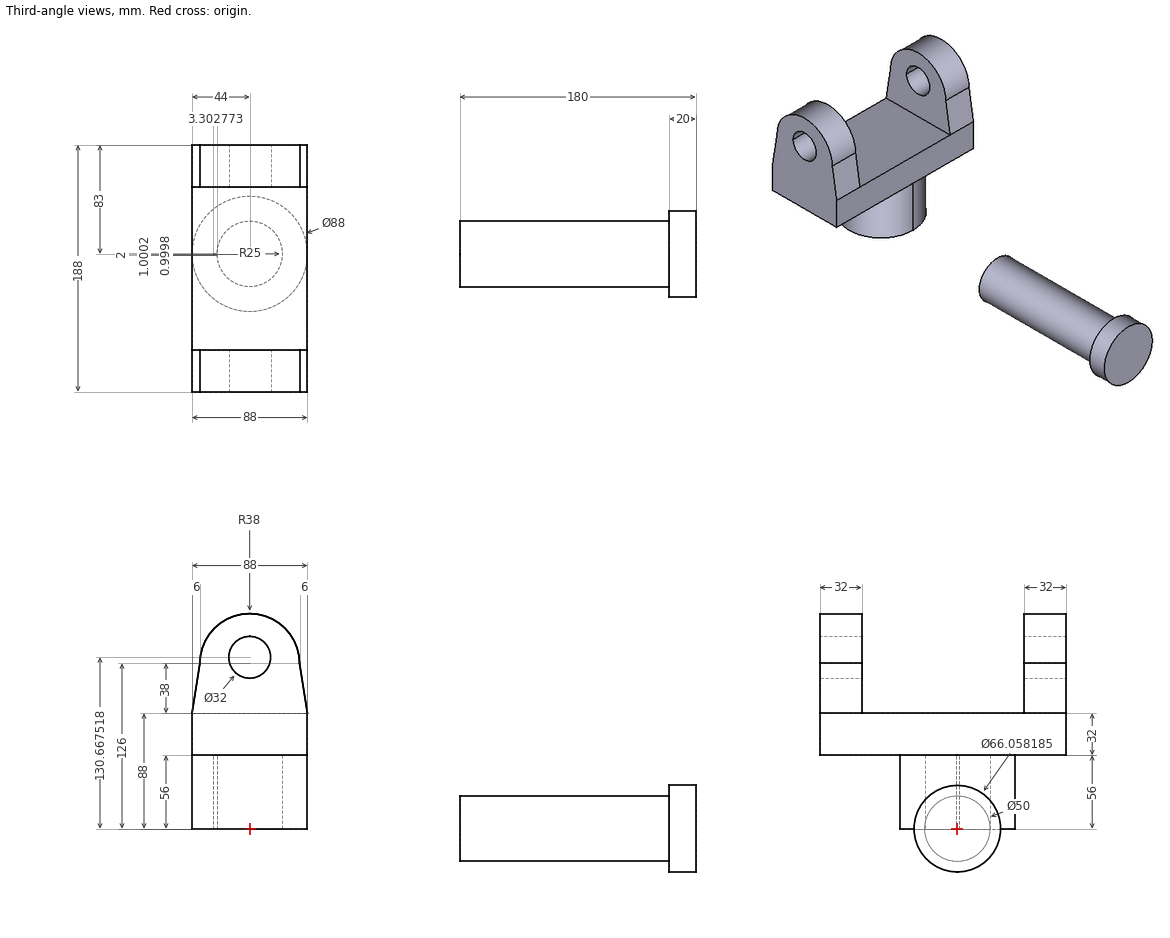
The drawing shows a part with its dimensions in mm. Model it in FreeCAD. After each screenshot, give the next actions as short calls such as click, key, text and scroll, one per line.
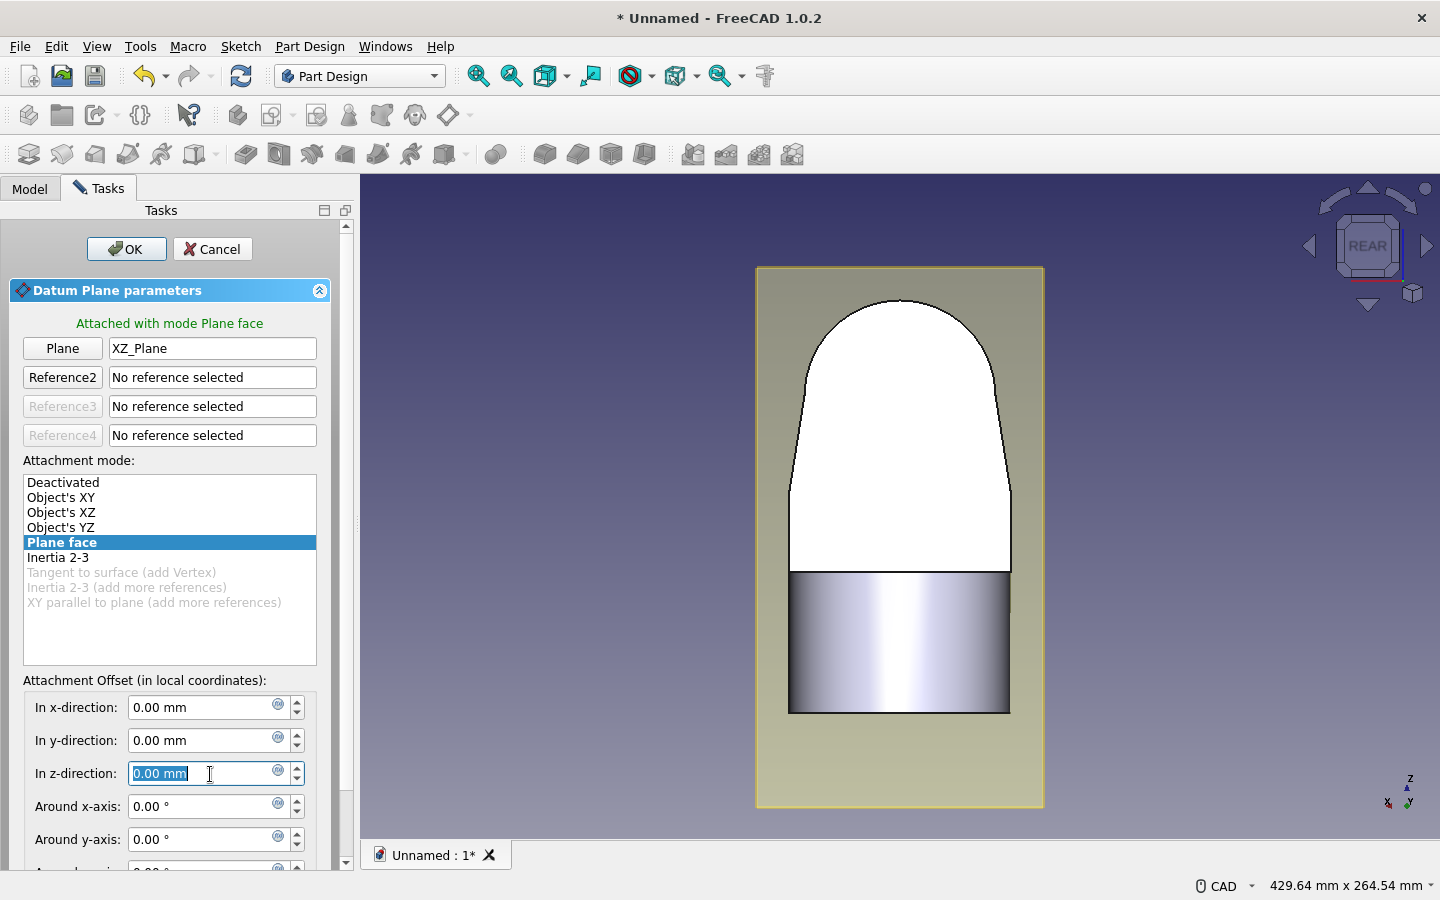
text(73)
key(Tab)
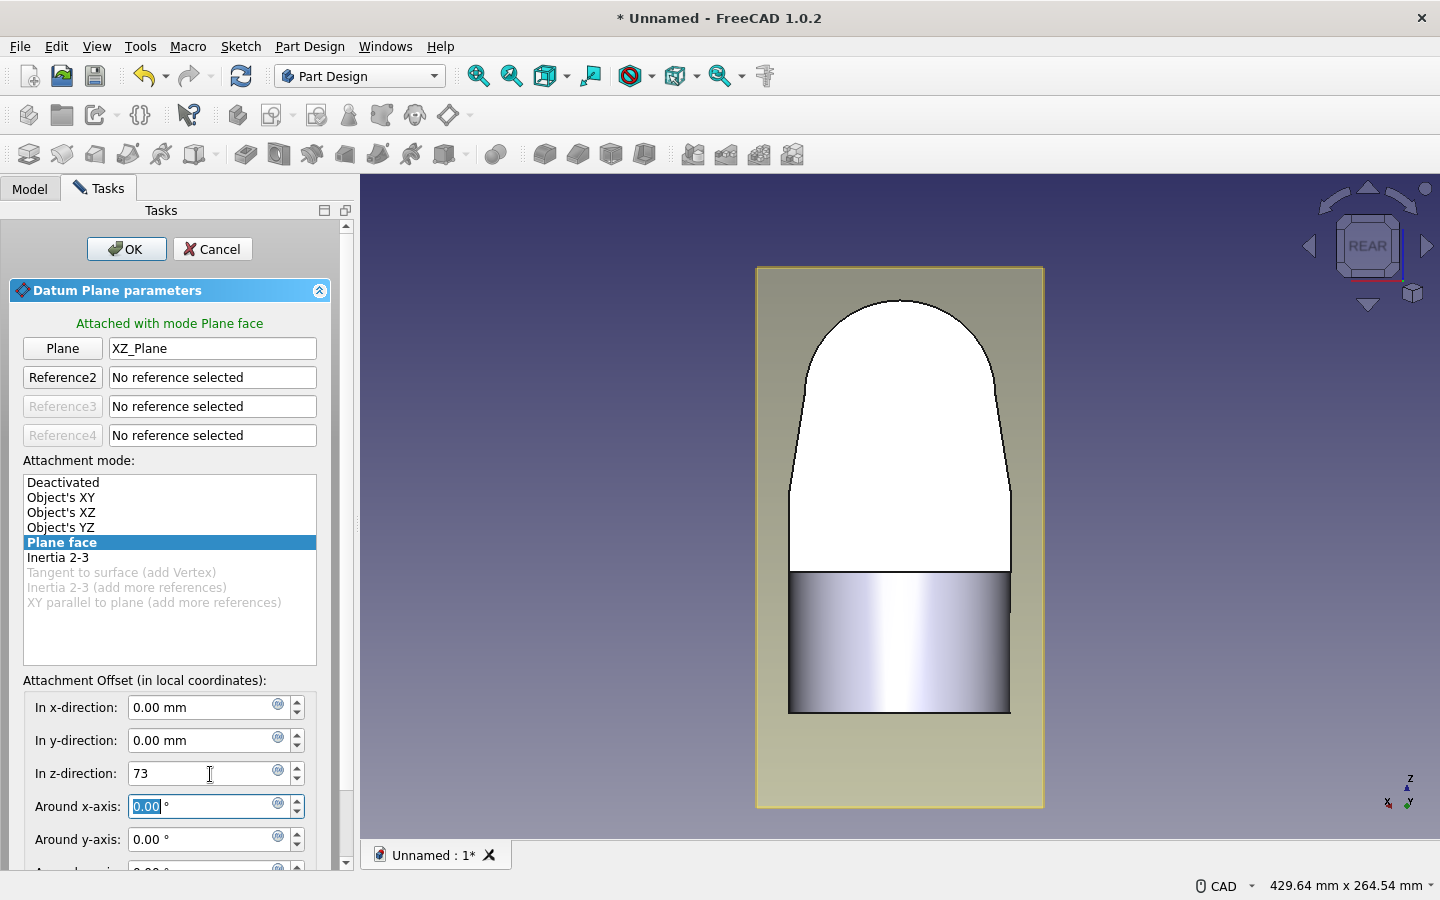
click(127, 249)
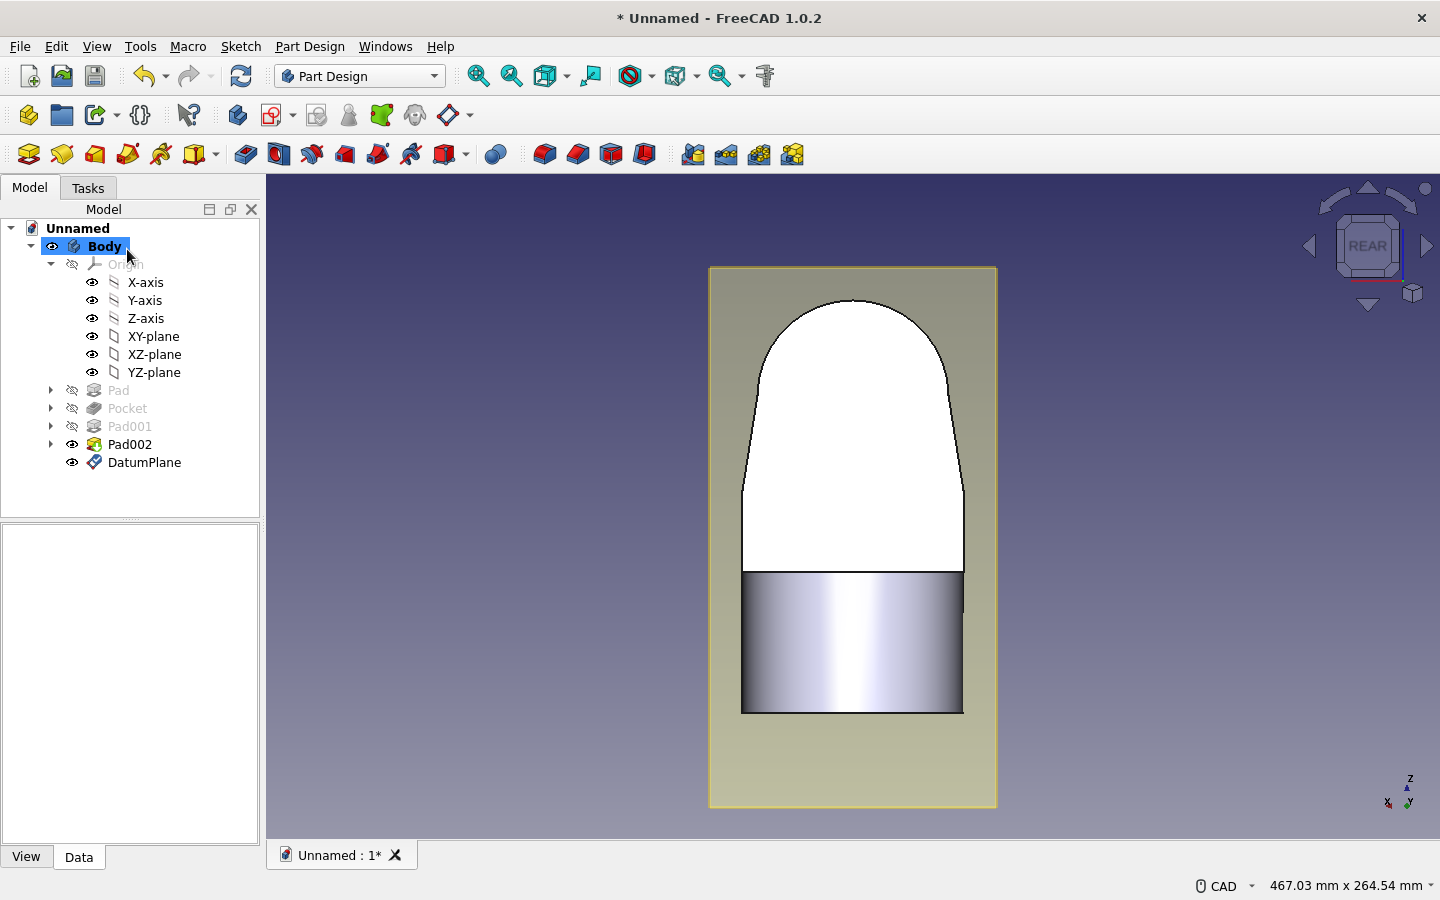
click(117, 462)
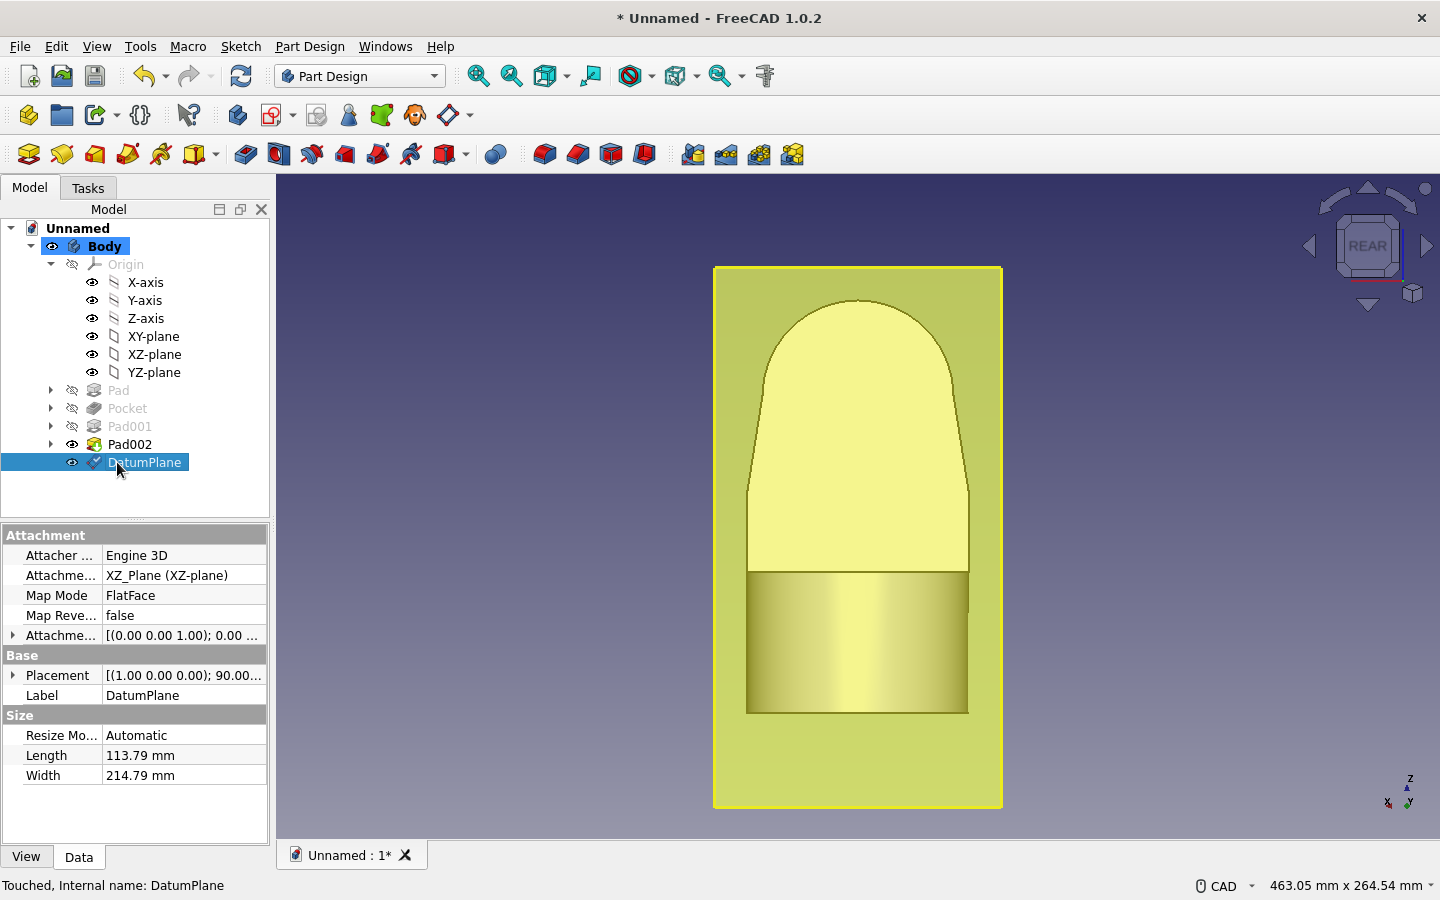
click(270, 116)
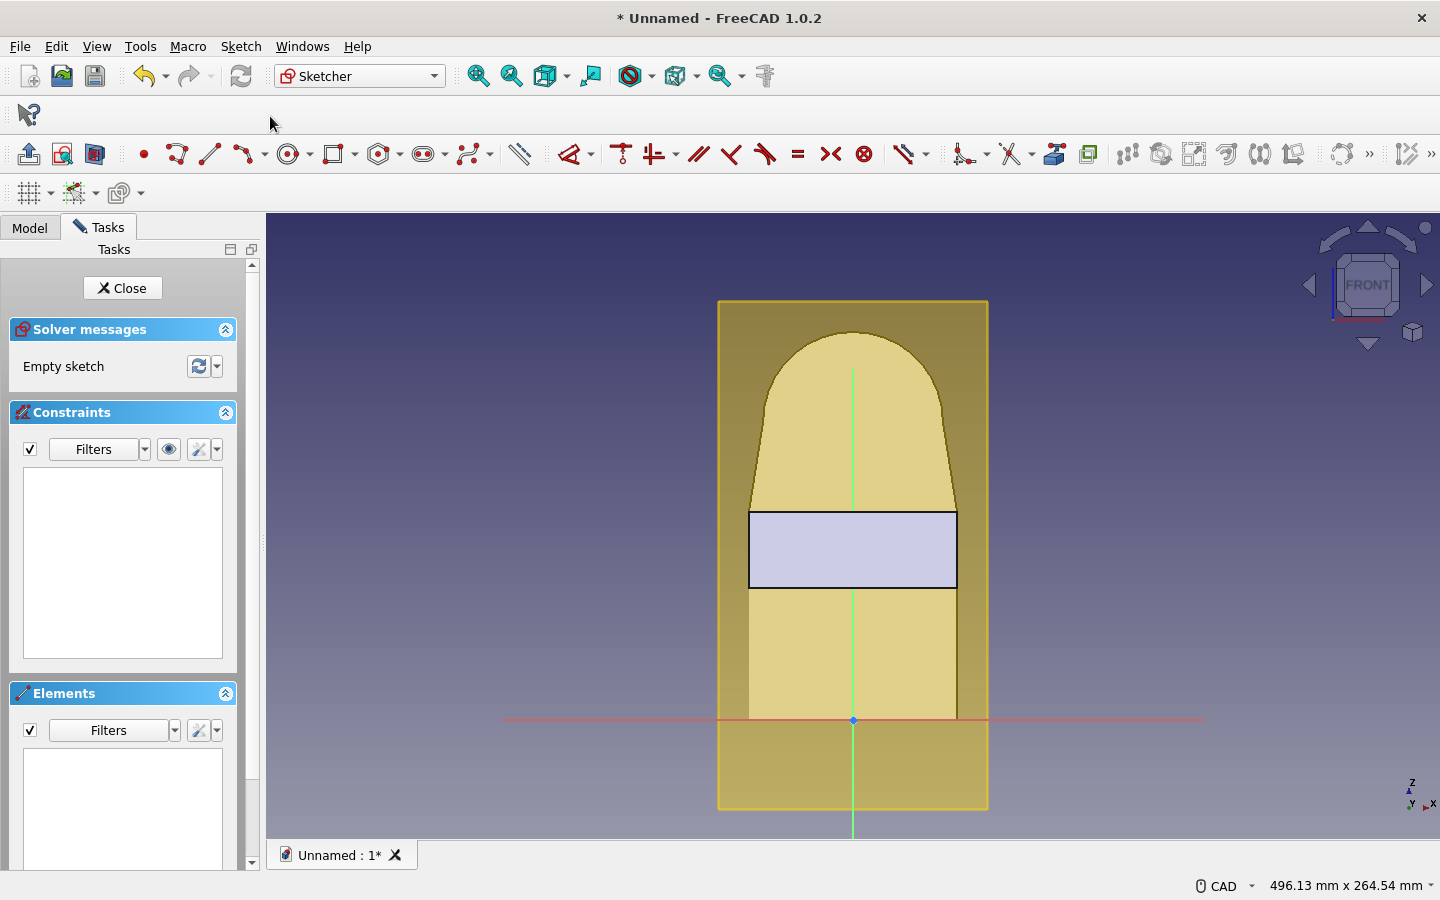
key(q)
key(s)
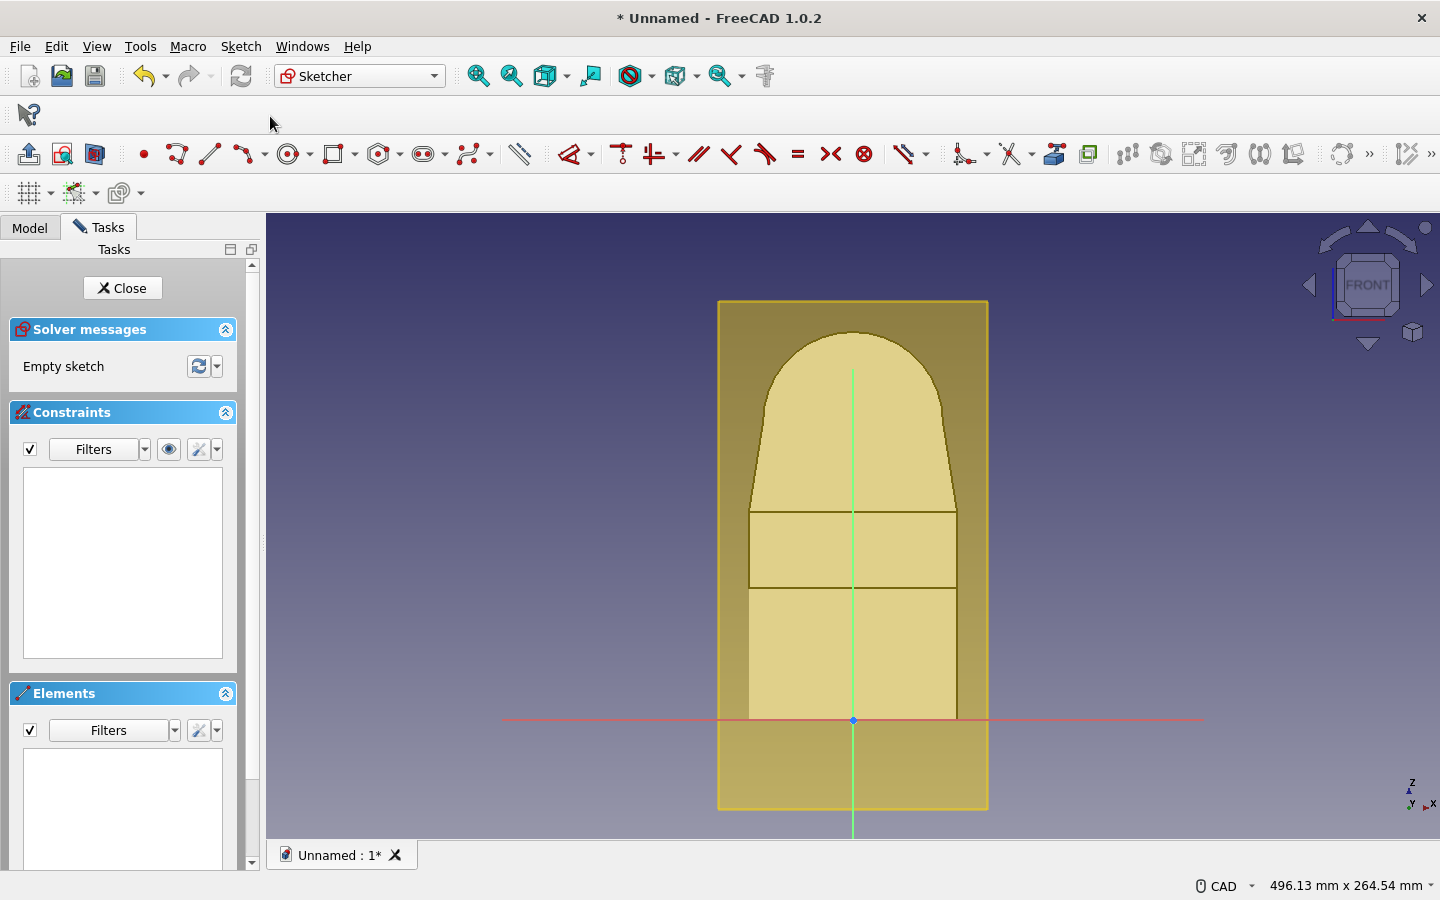
key(g)
key(m)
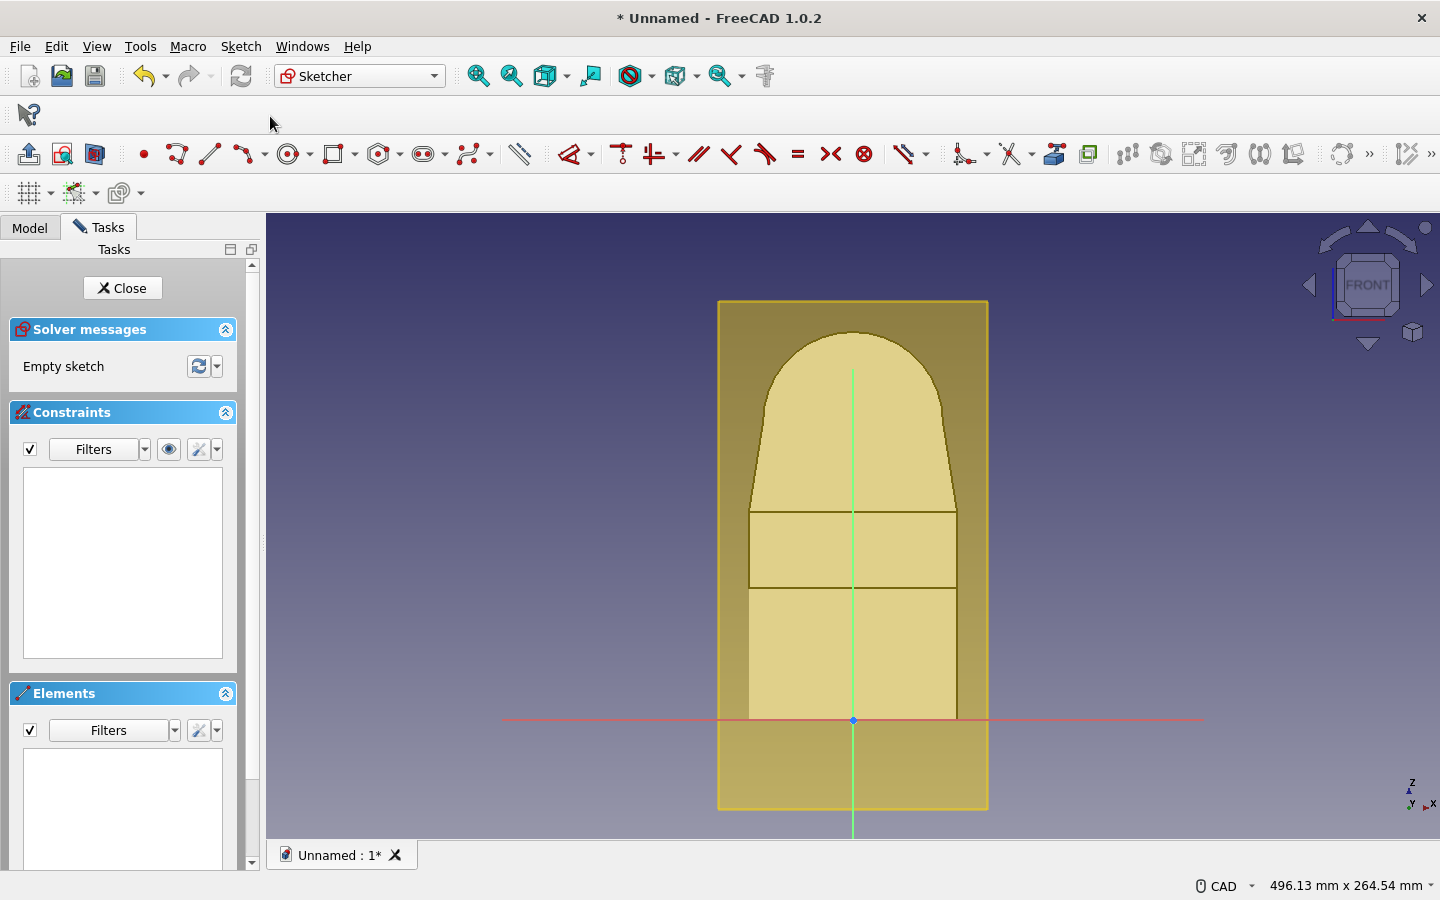
click(763, 422)
click(749, 512)
click(957, 512)
click(943, 422)
right_click(943, 422)